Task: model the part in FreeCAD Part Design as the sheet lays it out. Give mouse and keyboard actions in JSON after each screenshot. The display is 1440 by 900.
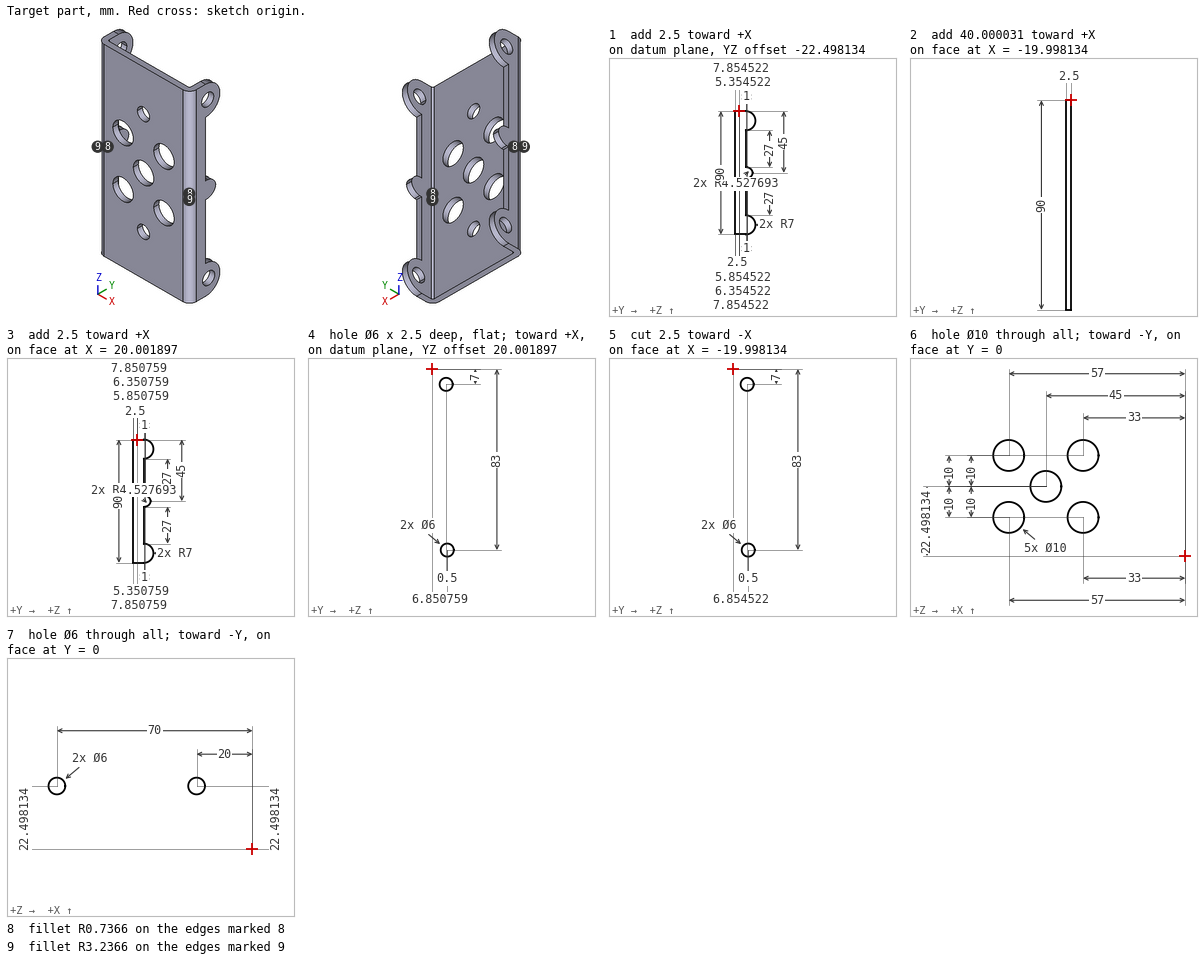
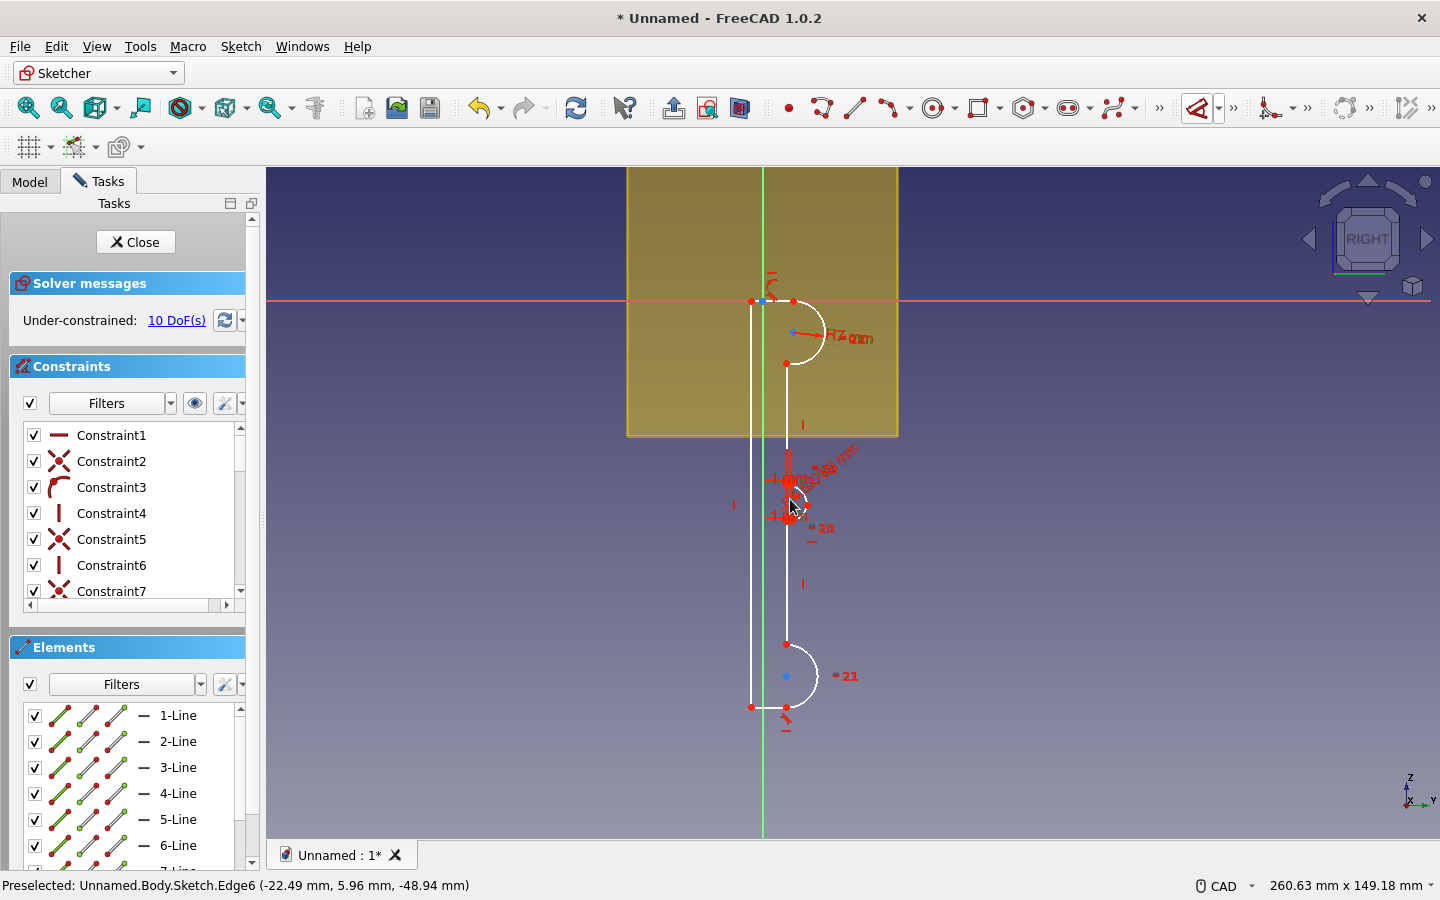
{"action": "left_click", "coordinate": [751, 586]}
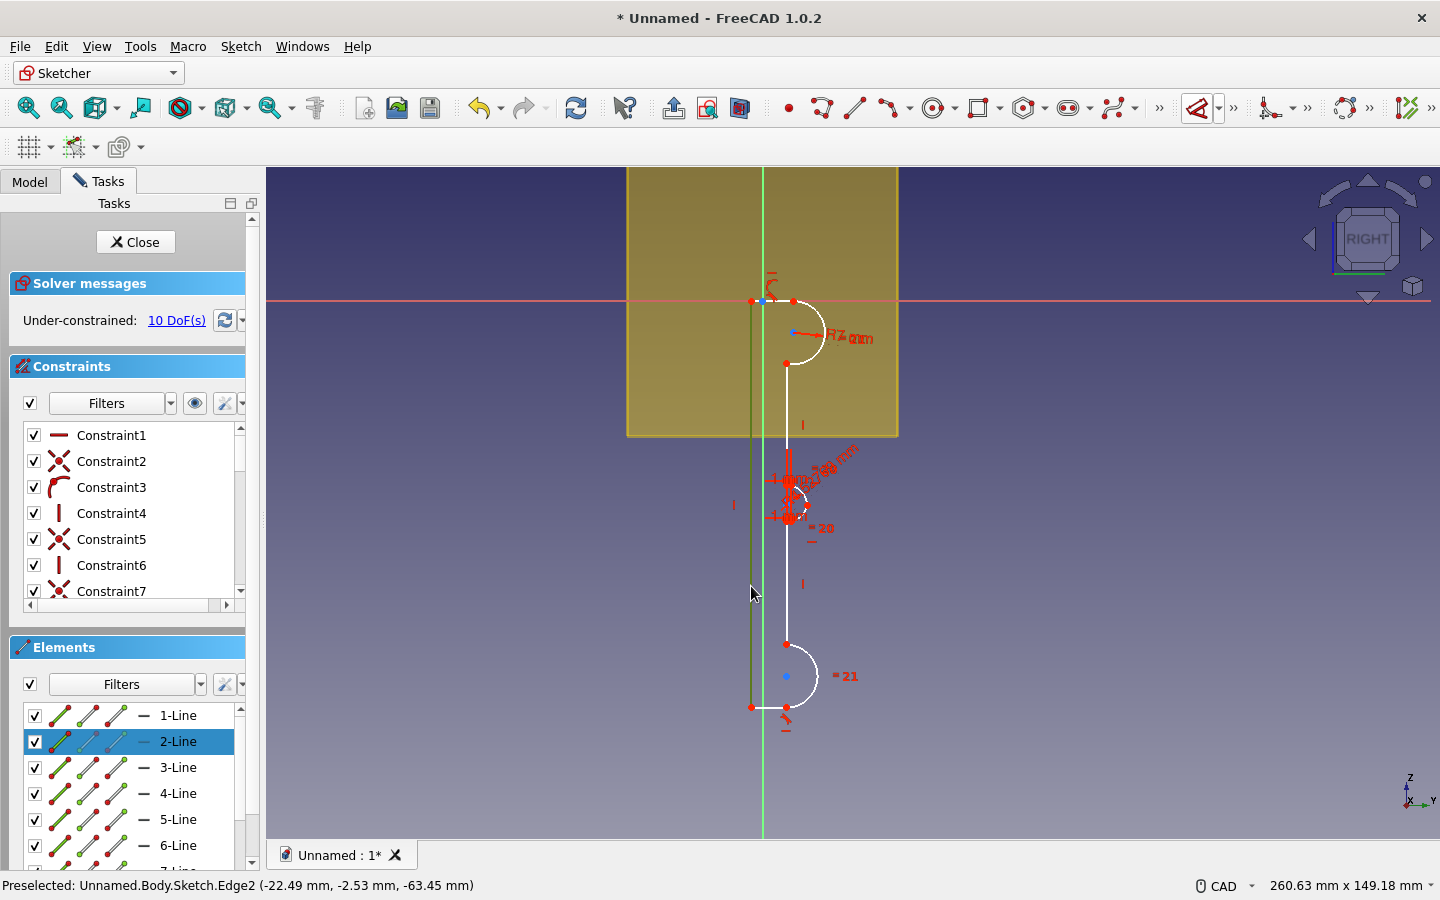
{"action": "left_click", "coordinate": [1218, 108]}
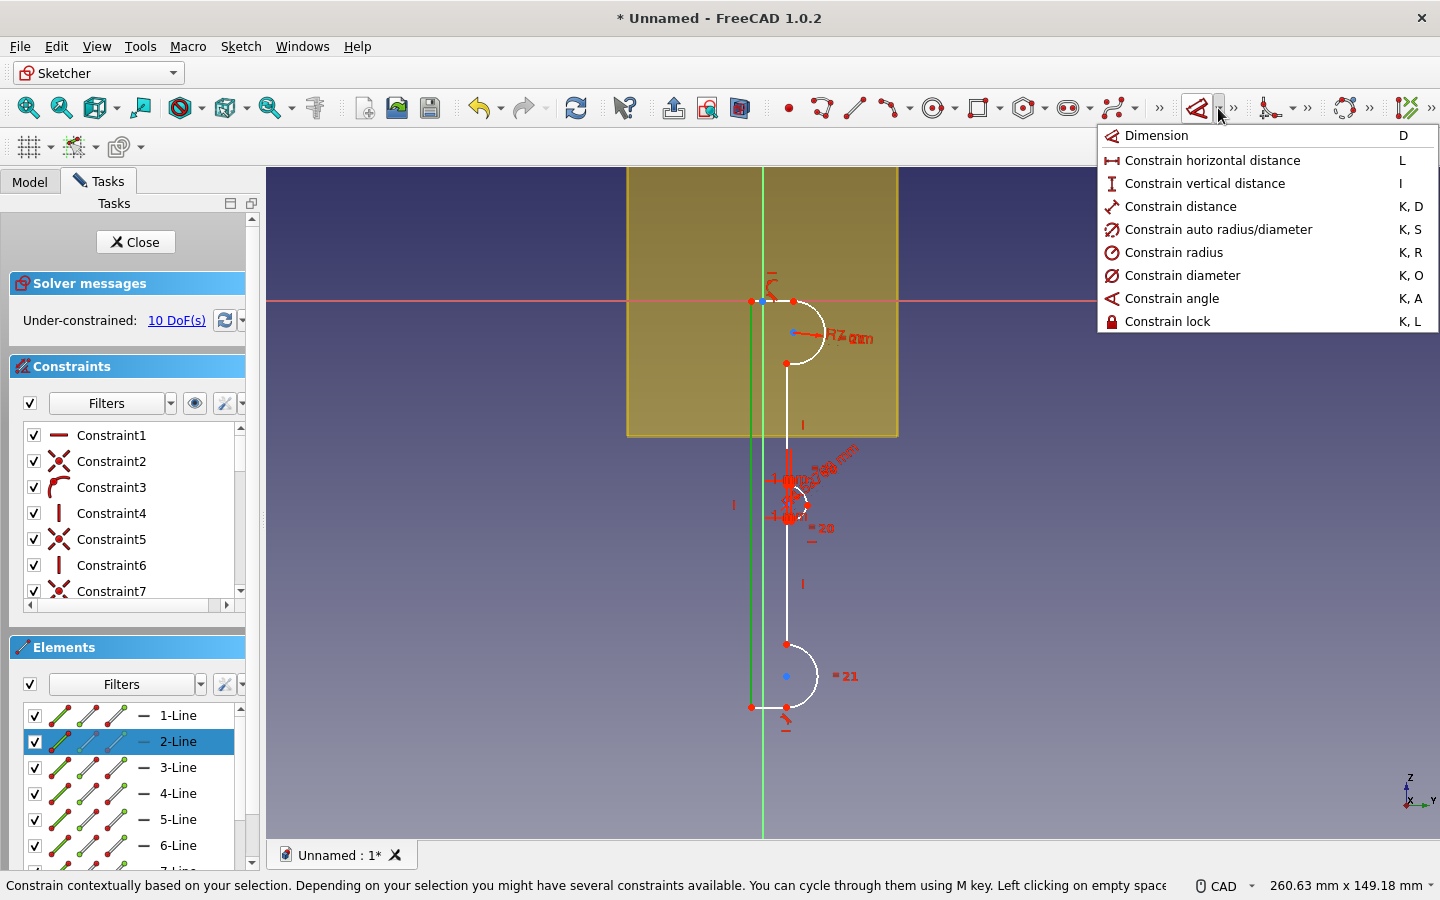
{"action": "left_click", "coordinate": [1268, 184]}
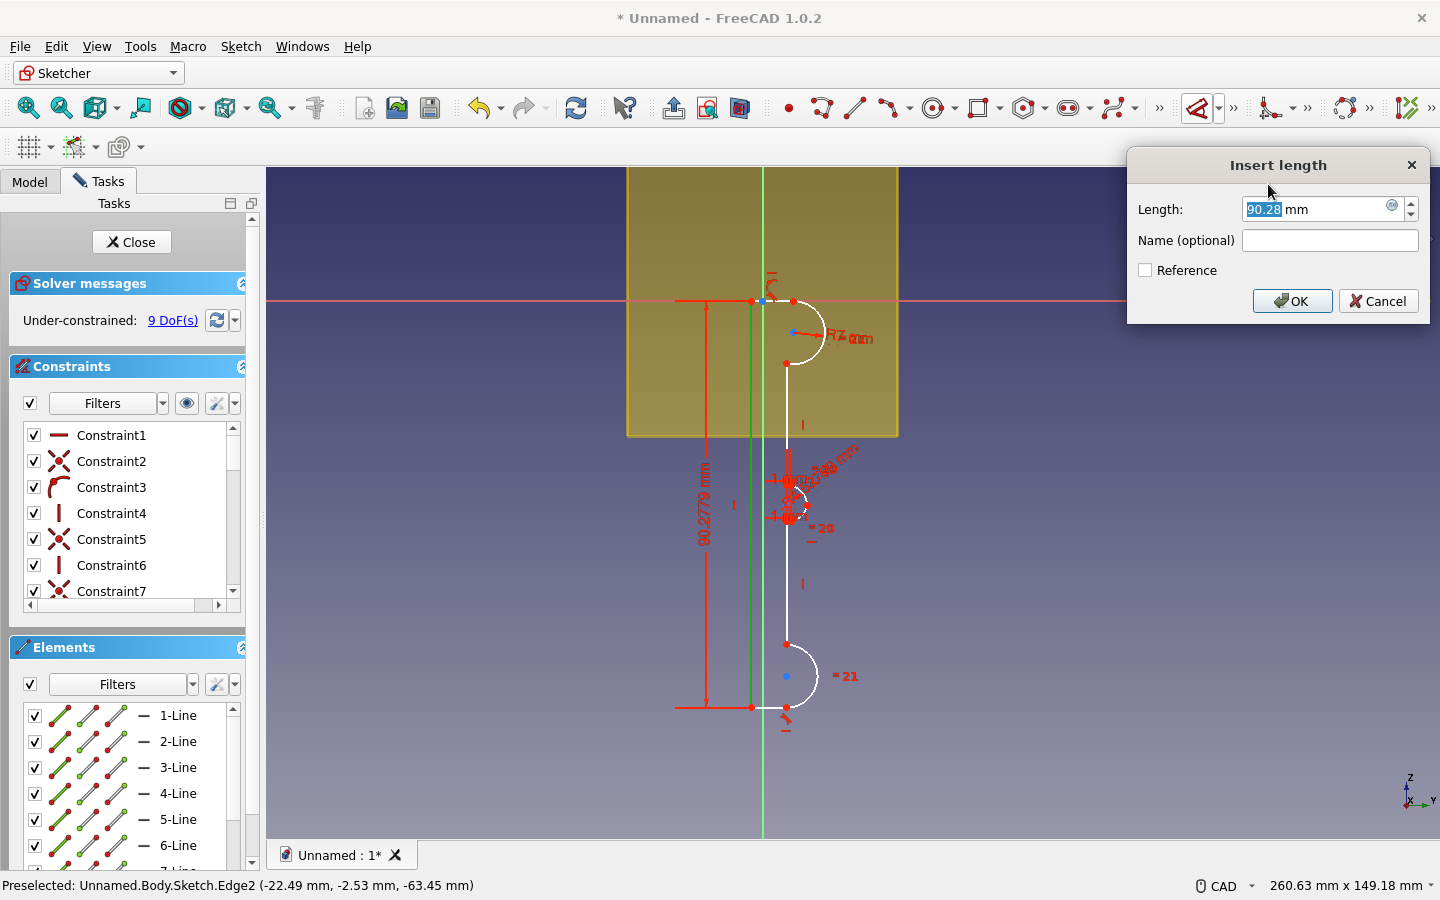
{"action": "type", "text": "90"}
{"action": "key", "text": "Return"}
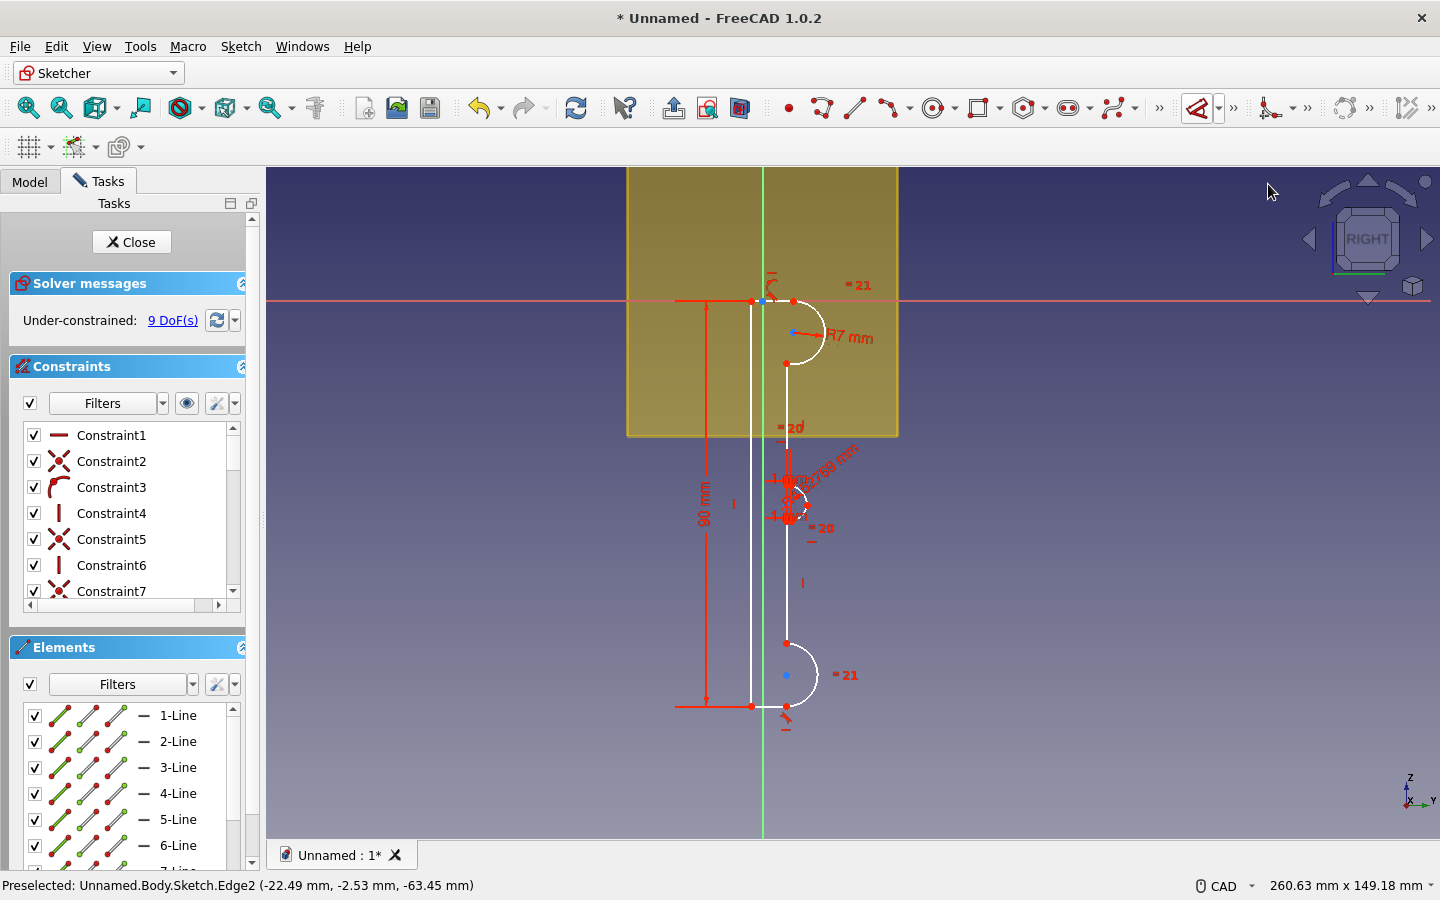
{"action": "left_click", "coordinate": [787, 400]}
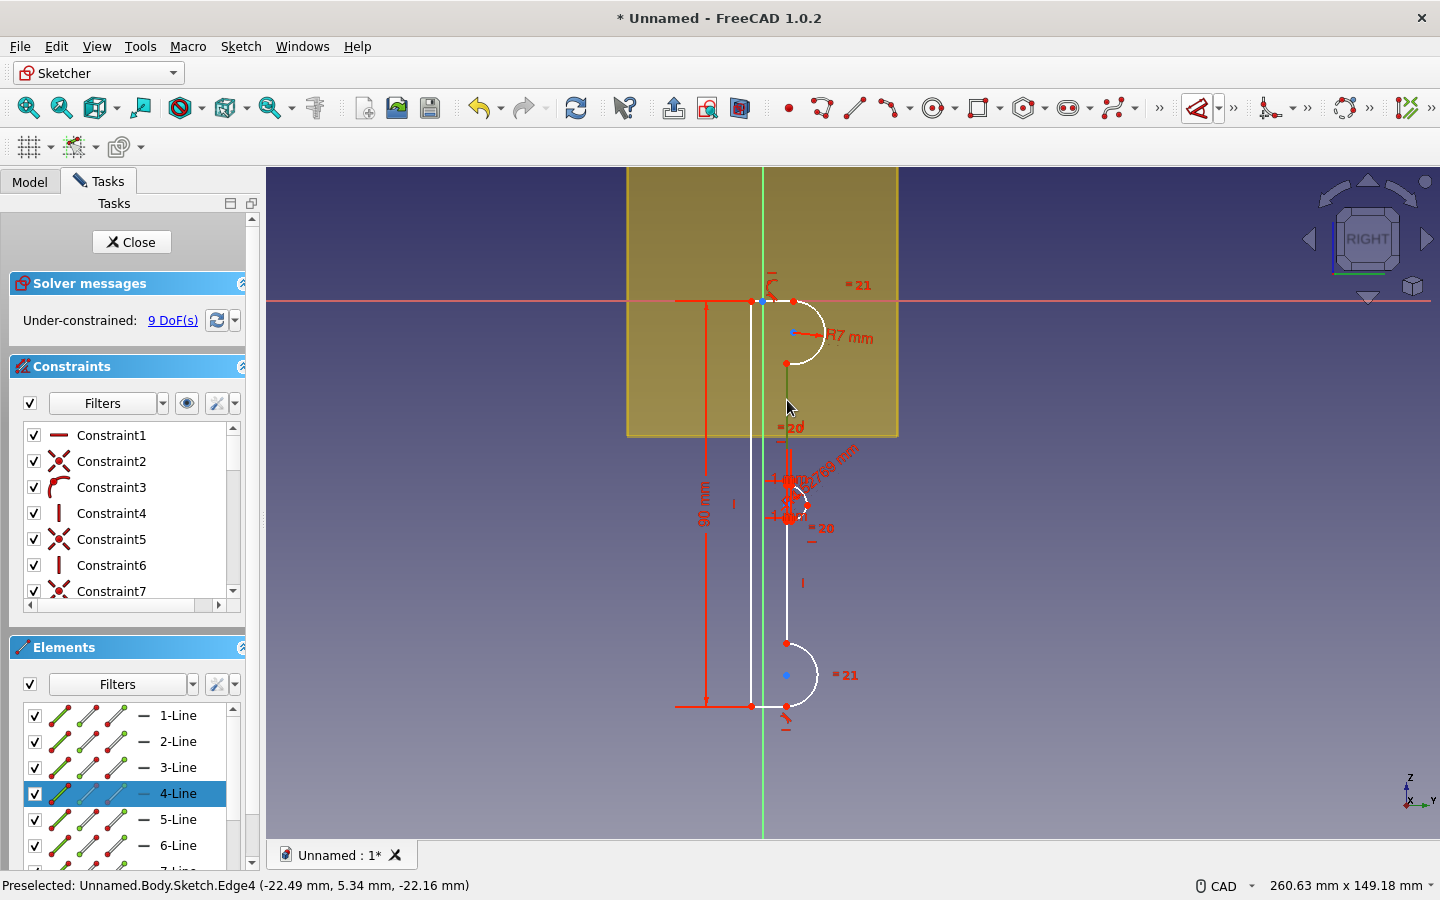
{"action": "key", "text": "i"}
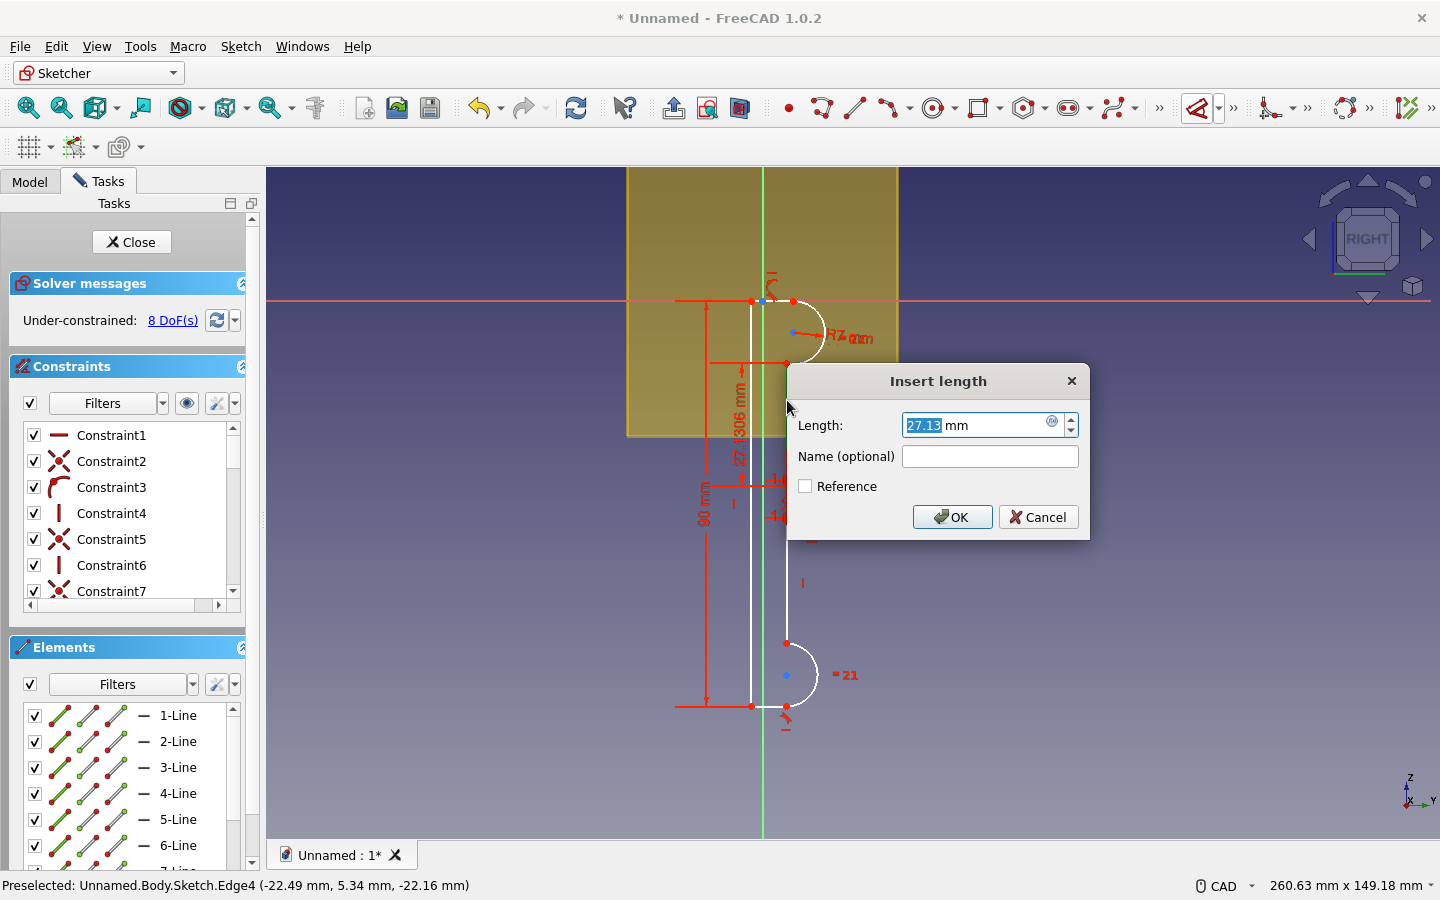
{"action": "type", "text": "27"}
{"action": "key", "text": "Return"}